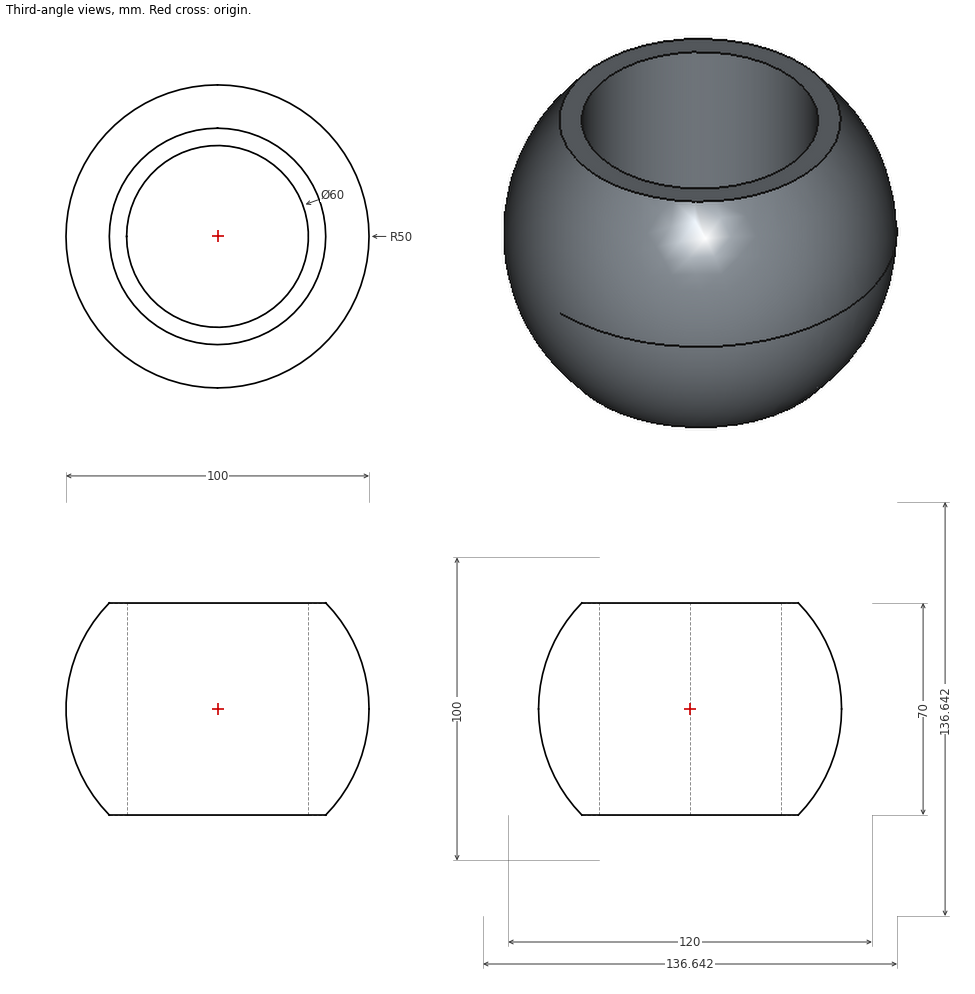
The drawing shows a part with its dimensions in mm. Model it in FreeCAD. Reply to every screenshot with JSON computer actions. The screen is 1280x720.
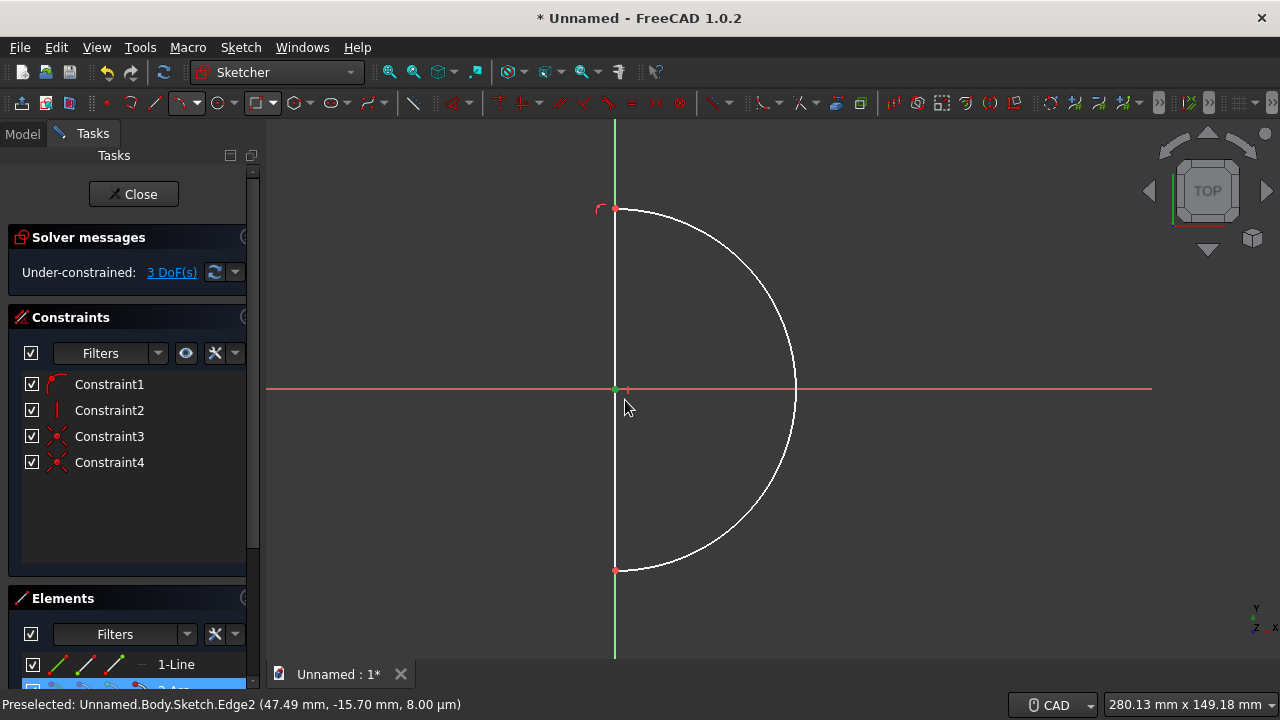
{"action": "left_click", "coordinate": [500, 104]}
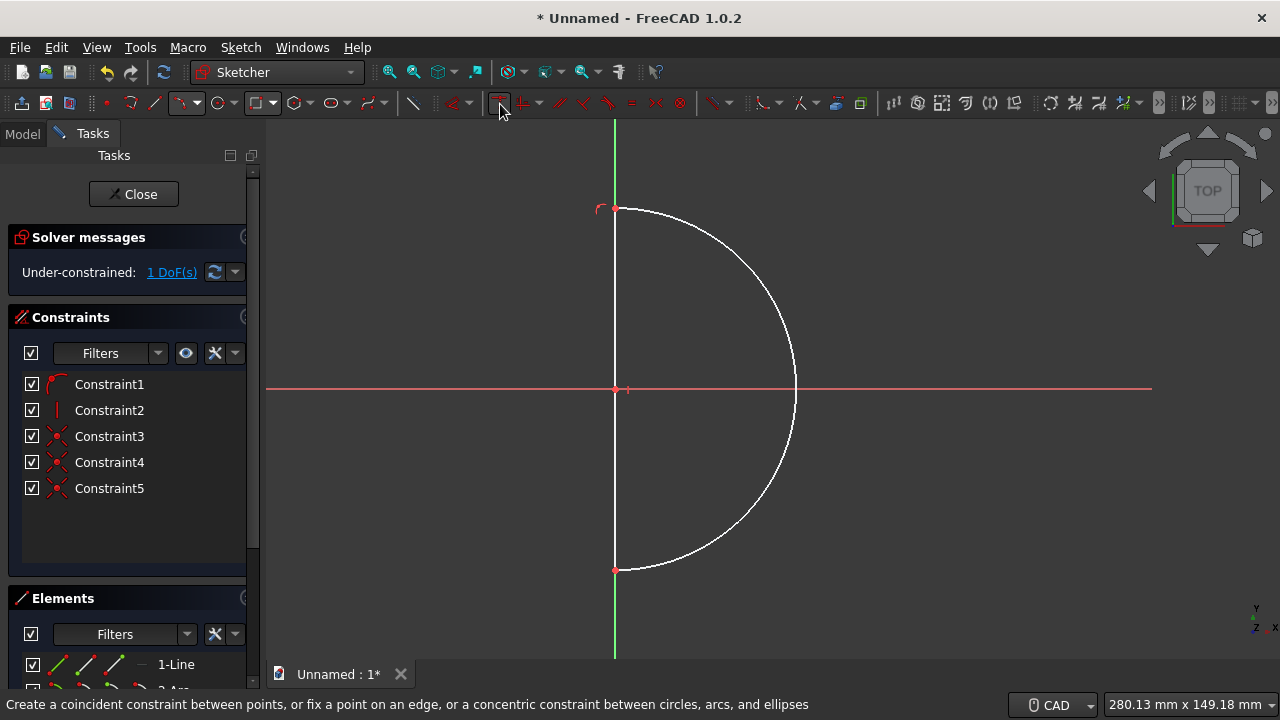
{"action": "left_click", "coordinate": [452, 104]}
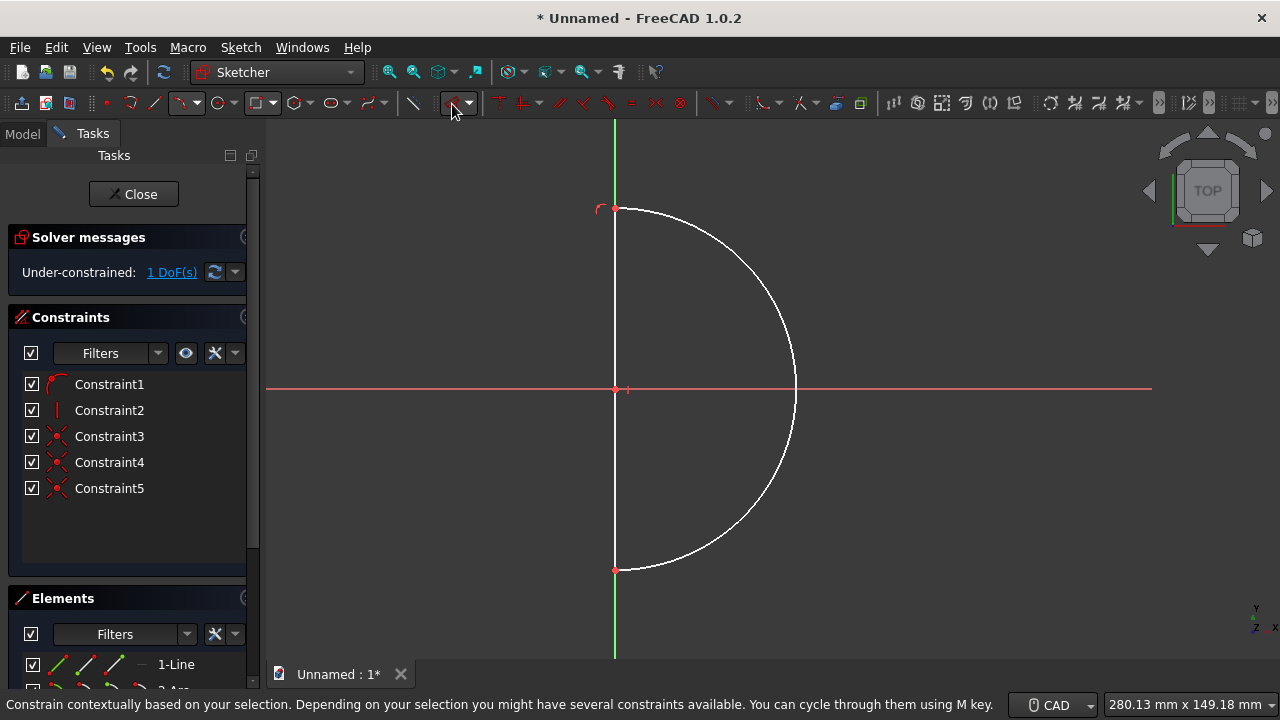
{"action": "left_click", "coordinate": [762, 496]}
{"action": "left_click", "coordinate": [788, 515]}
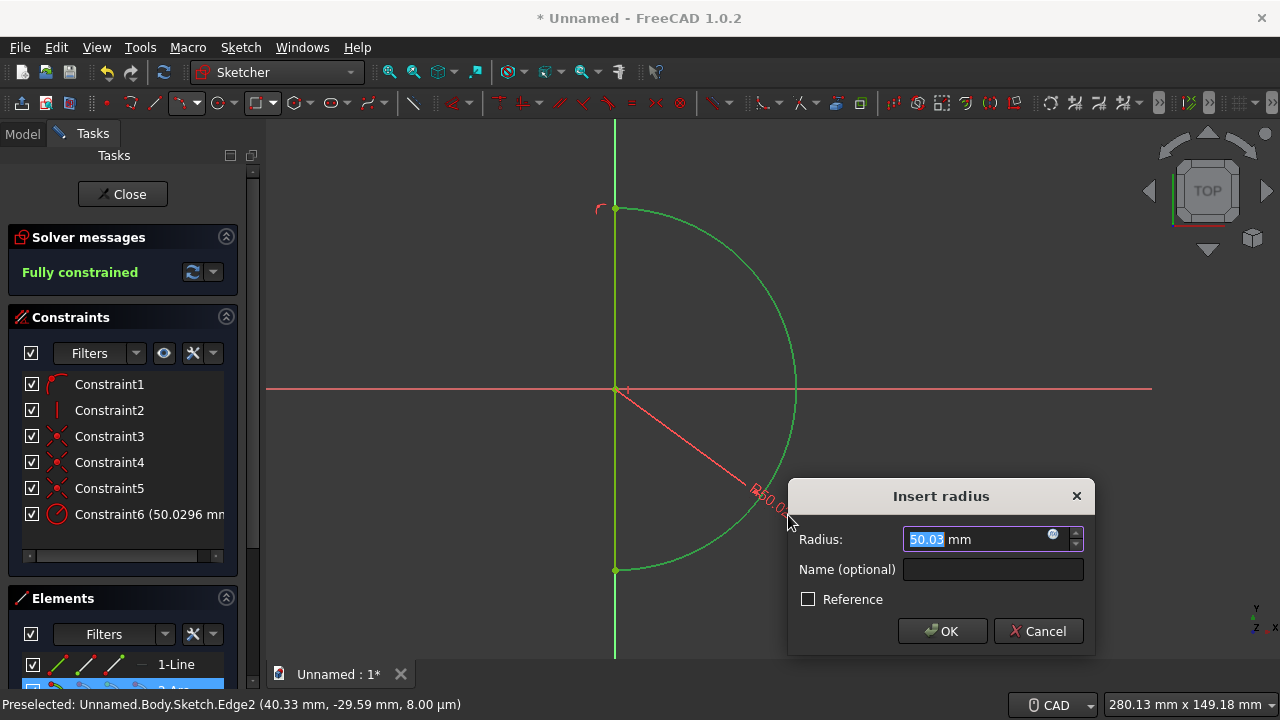
{"action": "type", "text": "50"}
{"action": "key", "text": "Return"}
{"action": "key", "text": "Escape"}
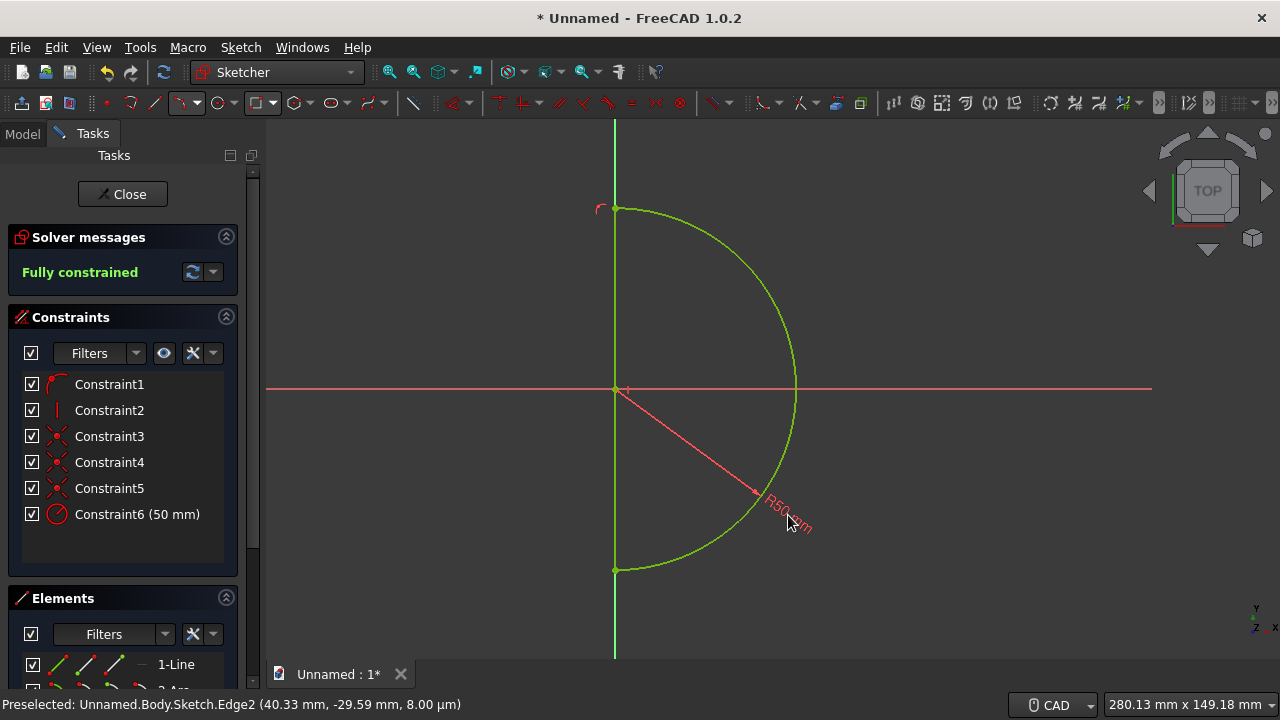
{"action": "left_click", "coordinate": [123, 194]}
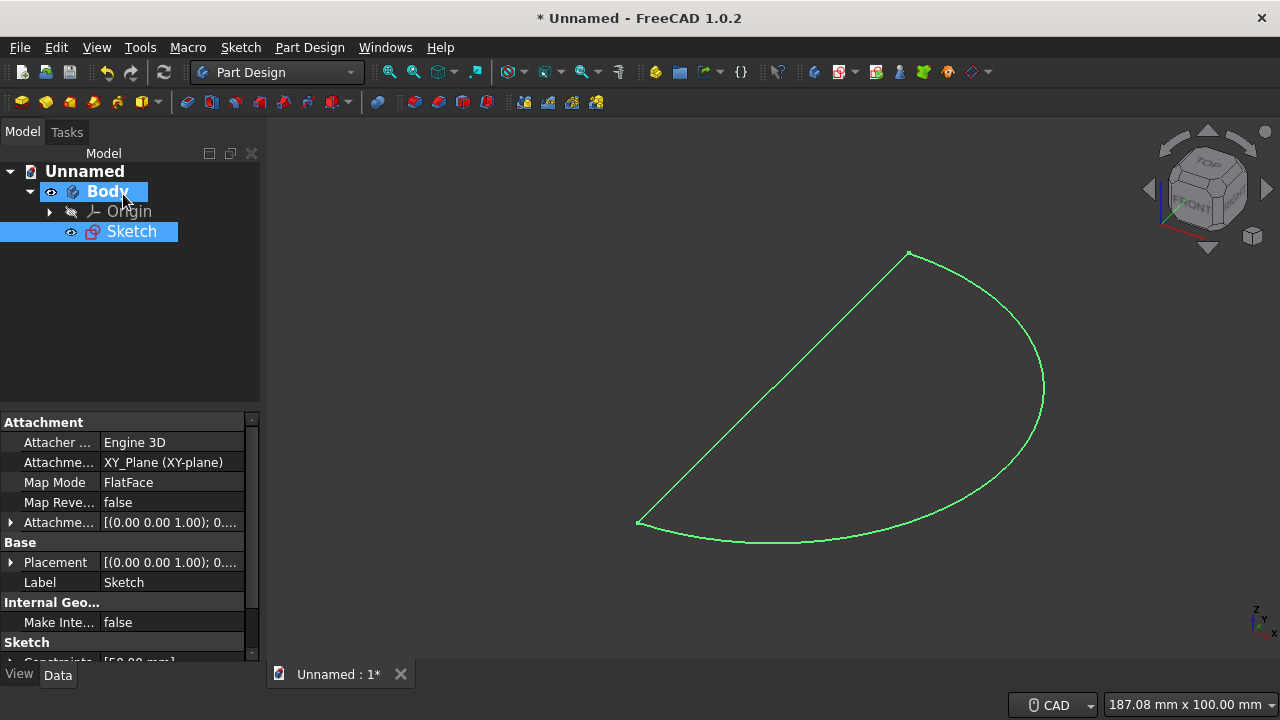
{"action": "left_click", "coordinate": [46, 102]}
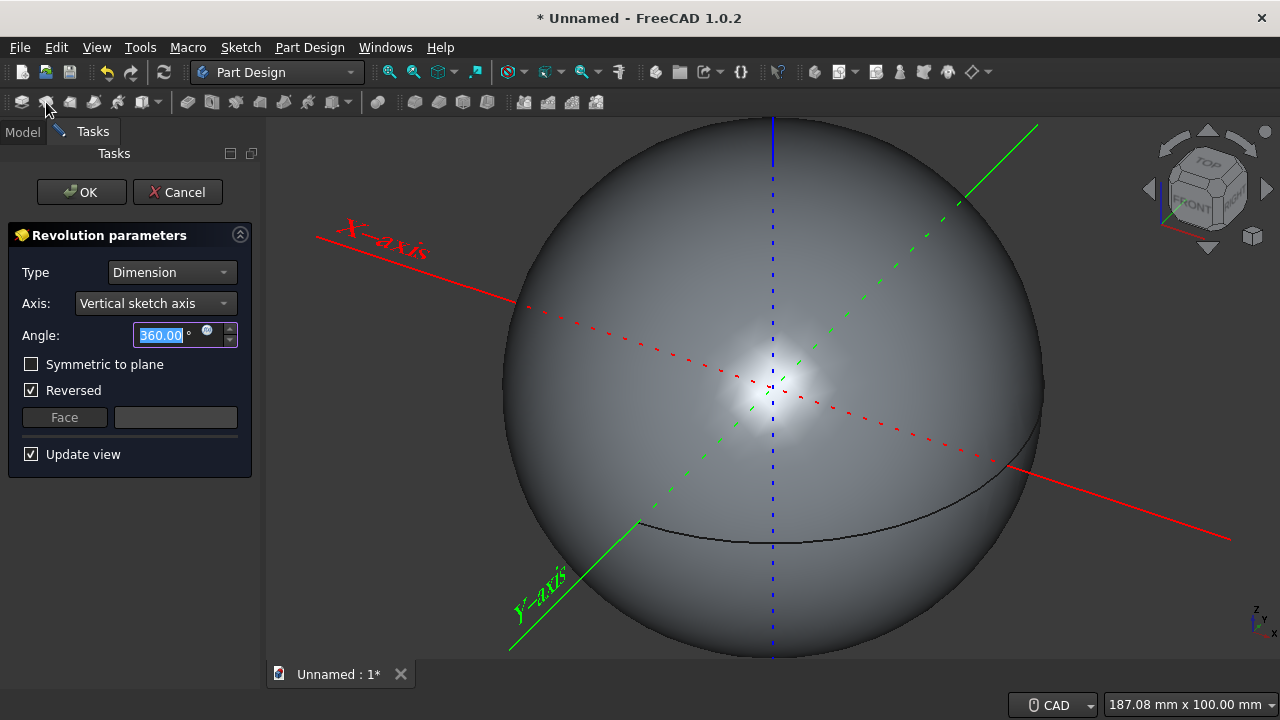
{"action": "left_click", "coordinate": [82, 192]}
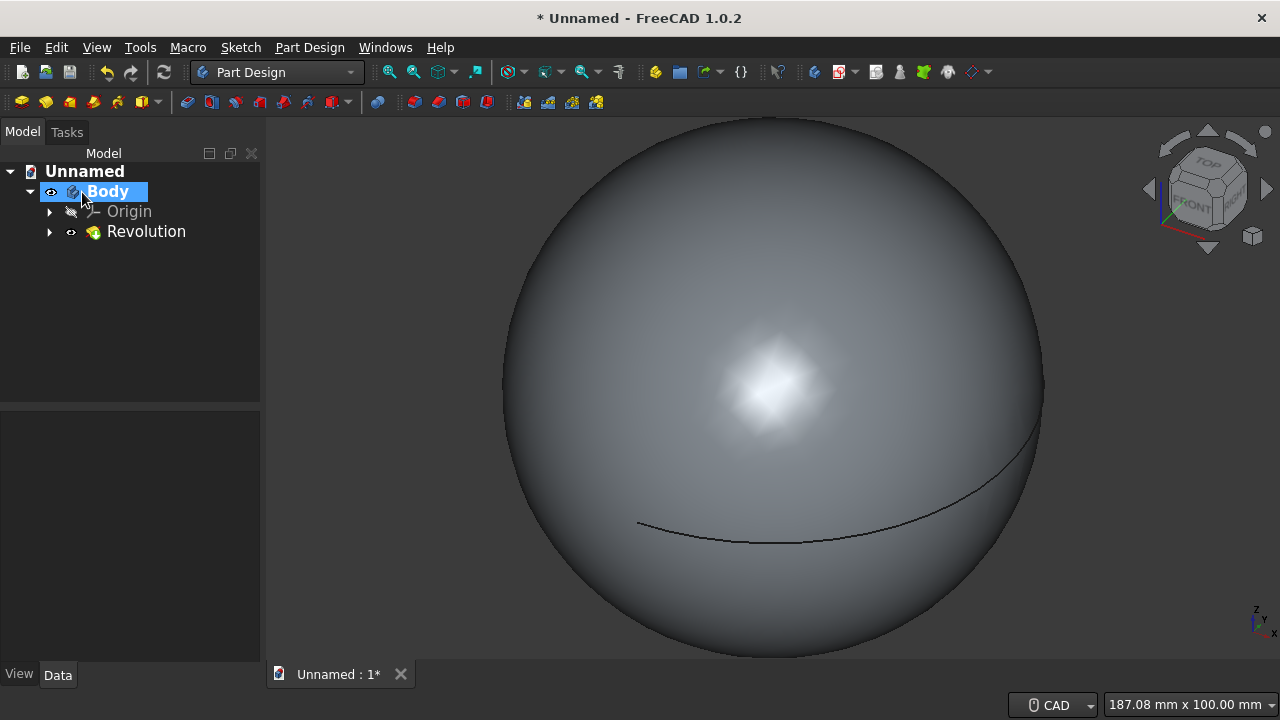
{"action": "left_click", "coordinate": [390, 72]}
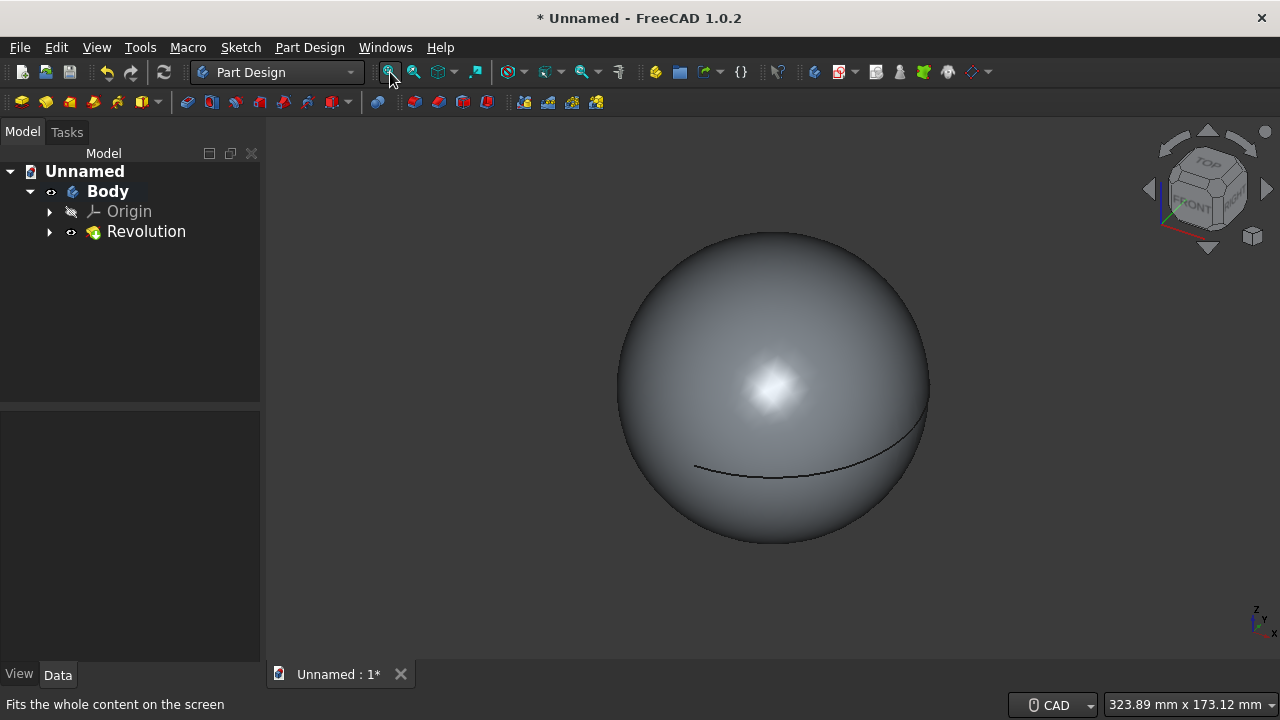
{"action": "left_click", "coordinate": [840, 72]}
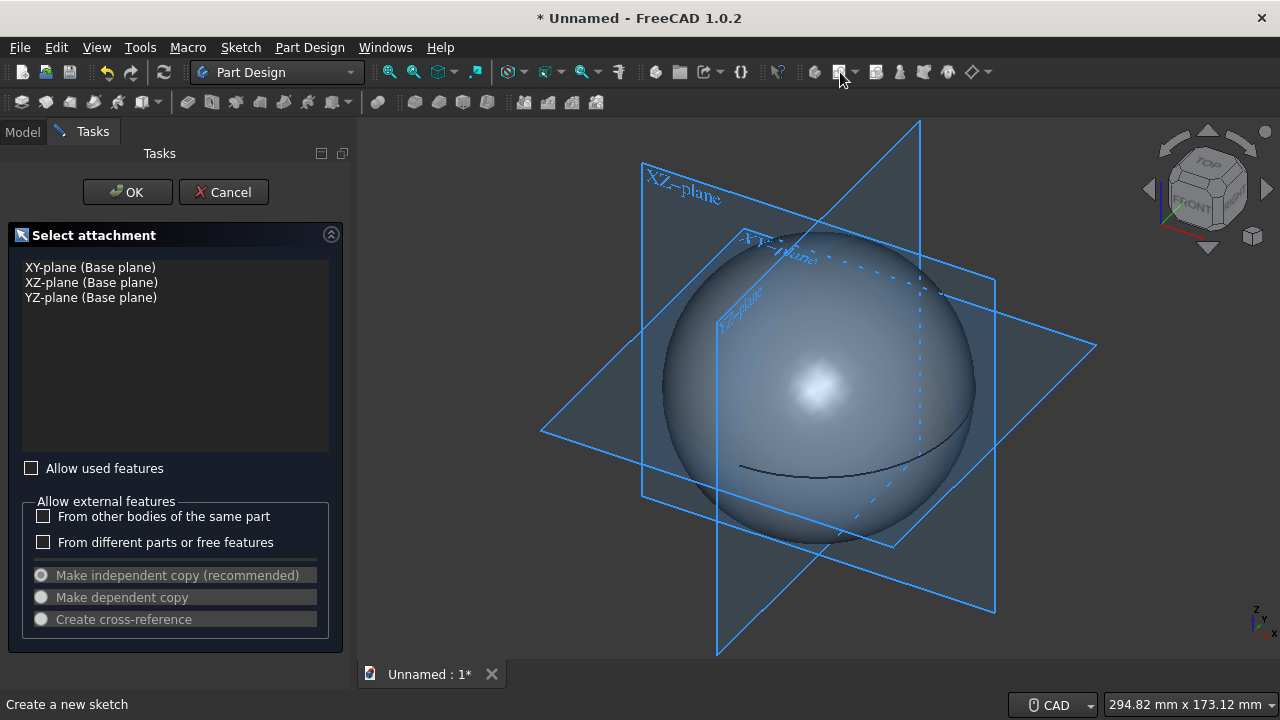
{"action": "left_click", "coordinate": [82, 268]}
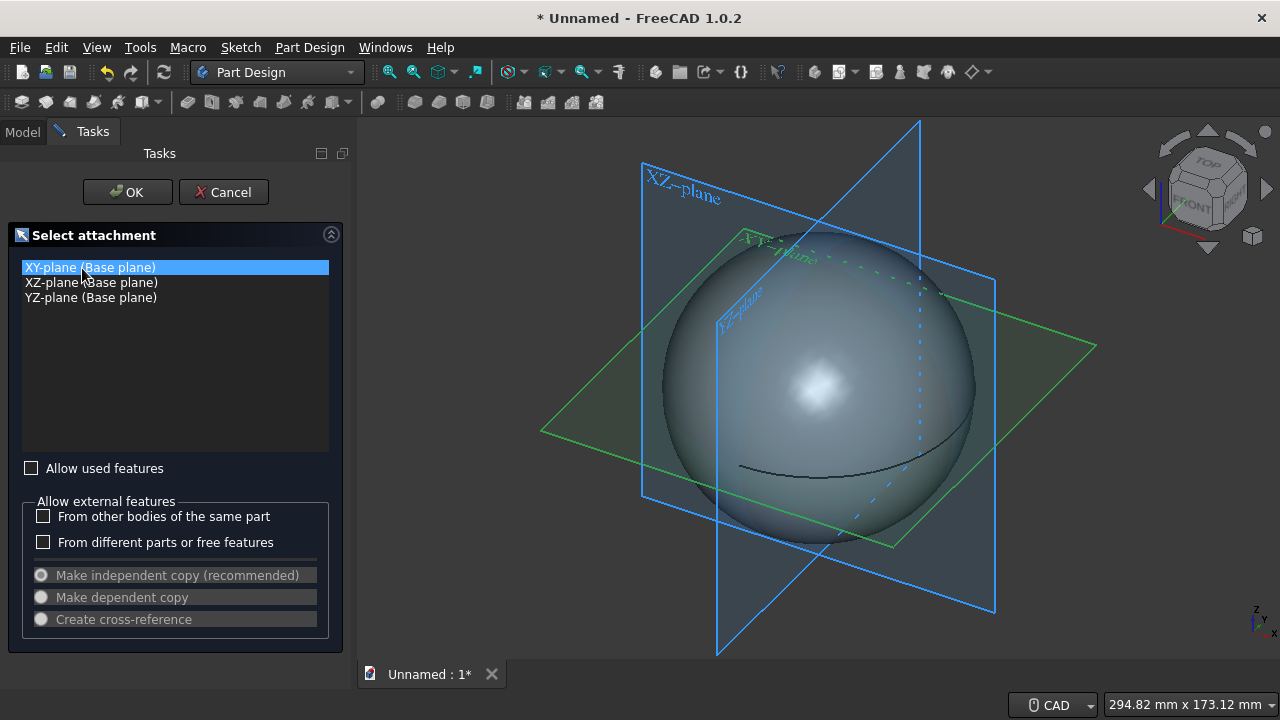
{"action": "left_click", "coordinate": [128, 192]}